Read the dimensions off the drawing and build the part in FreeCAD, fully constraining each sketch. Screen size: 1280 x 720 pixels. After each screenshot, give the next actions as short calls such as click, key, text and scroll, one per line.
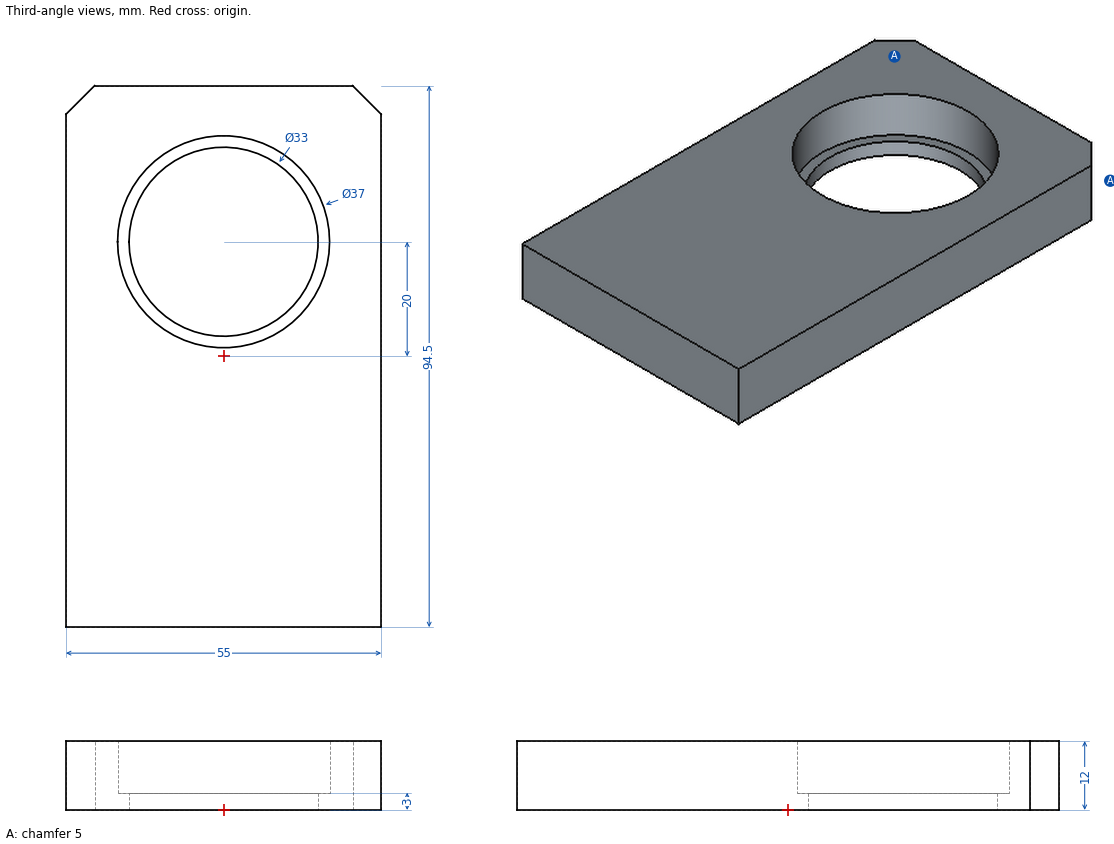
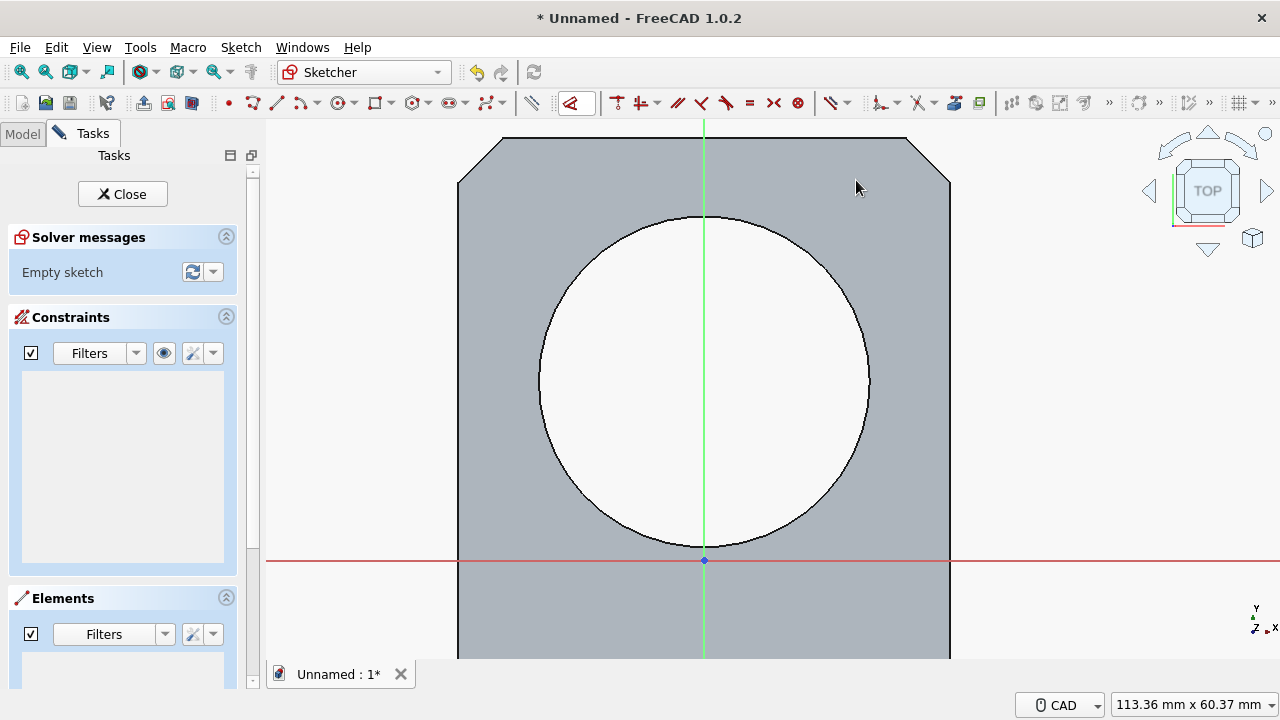
click(338, 104)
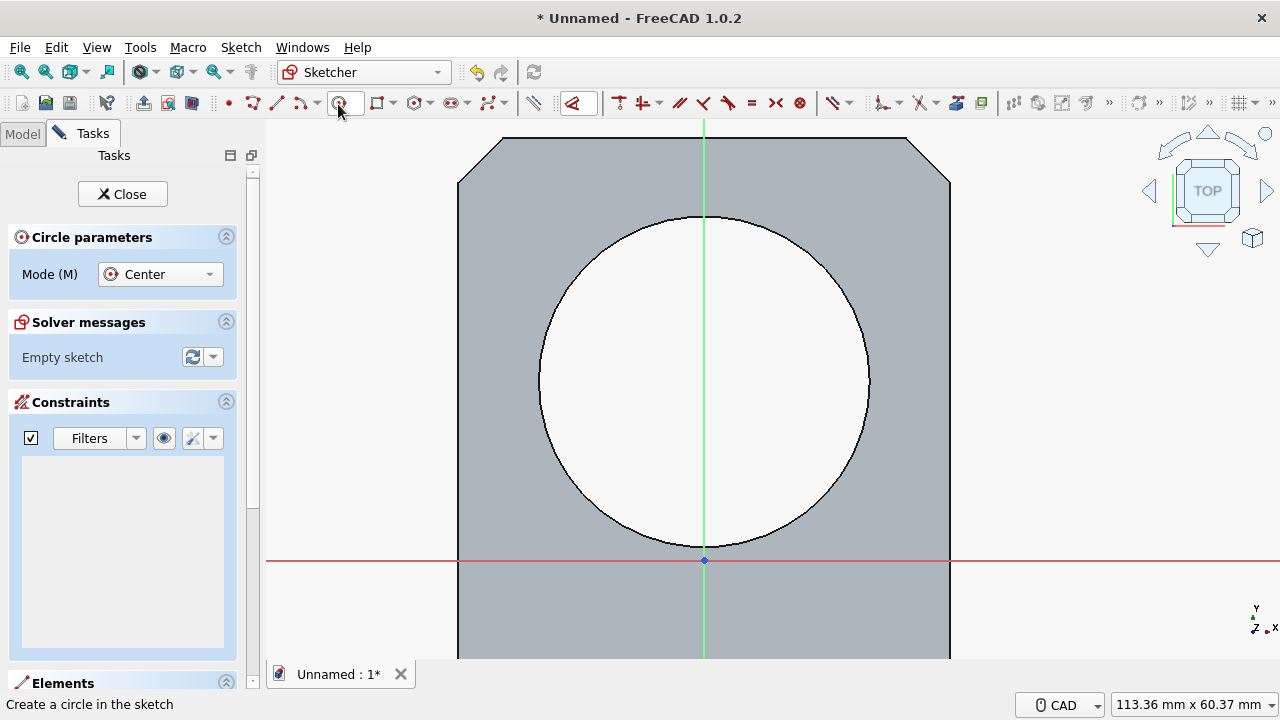
click(704, 382)
click(821, 265)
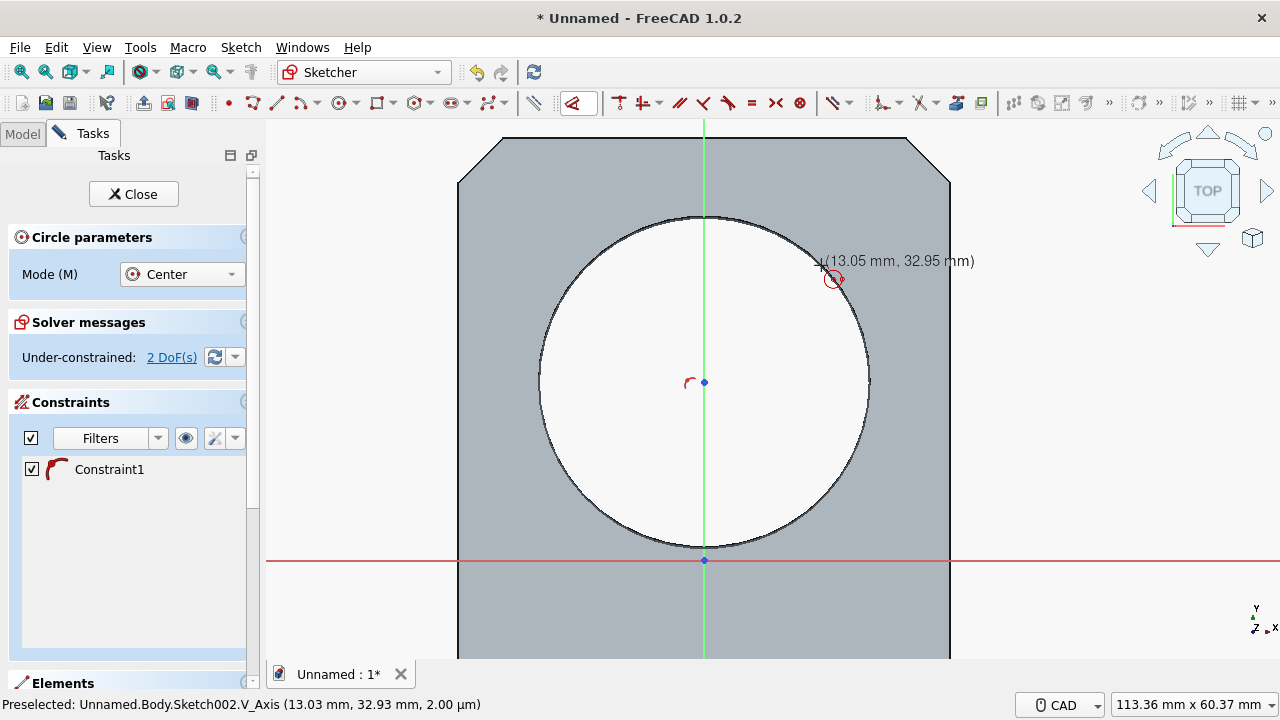
click(704, 383)
click(809, 277)
key(Escape)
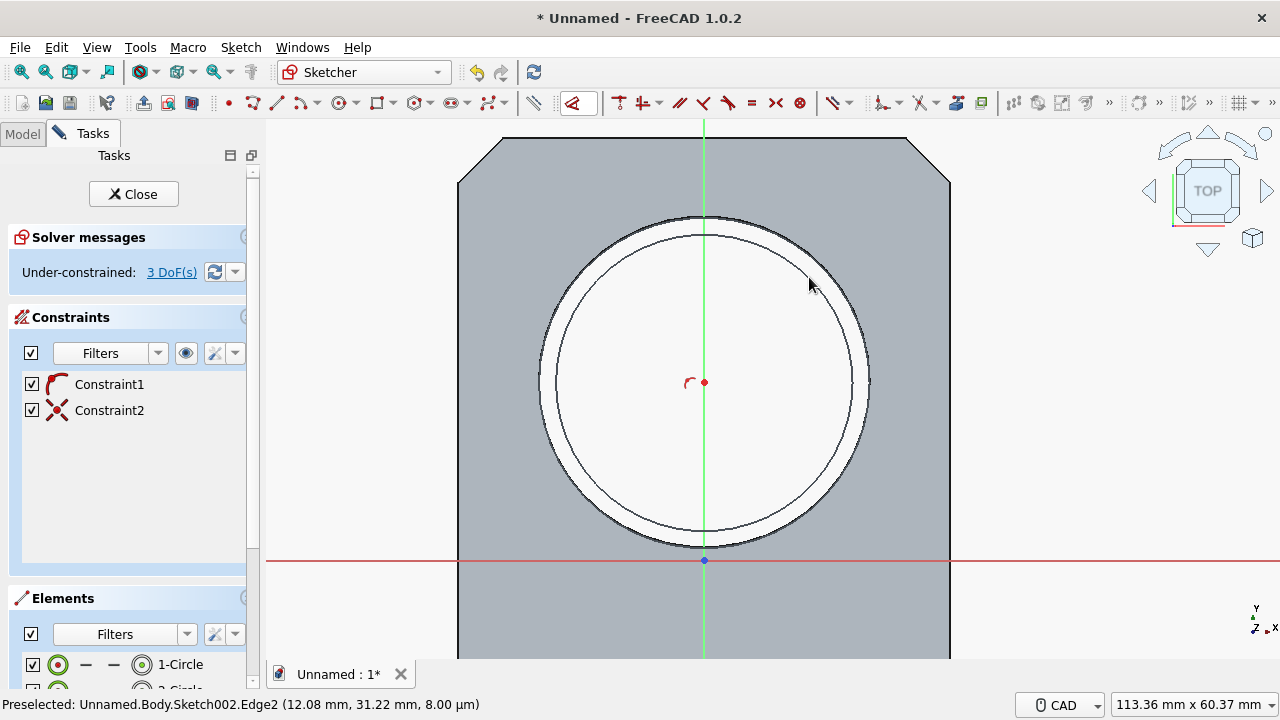
click(821, 266)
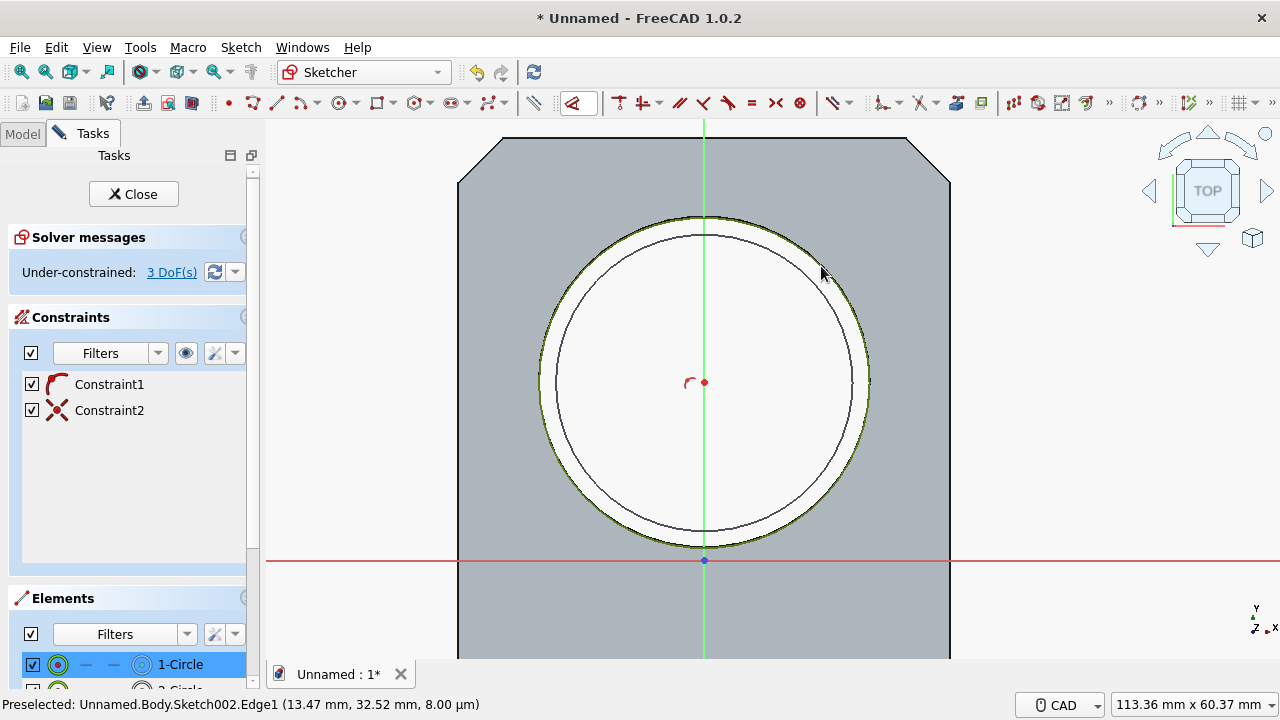
key(k)
key(o)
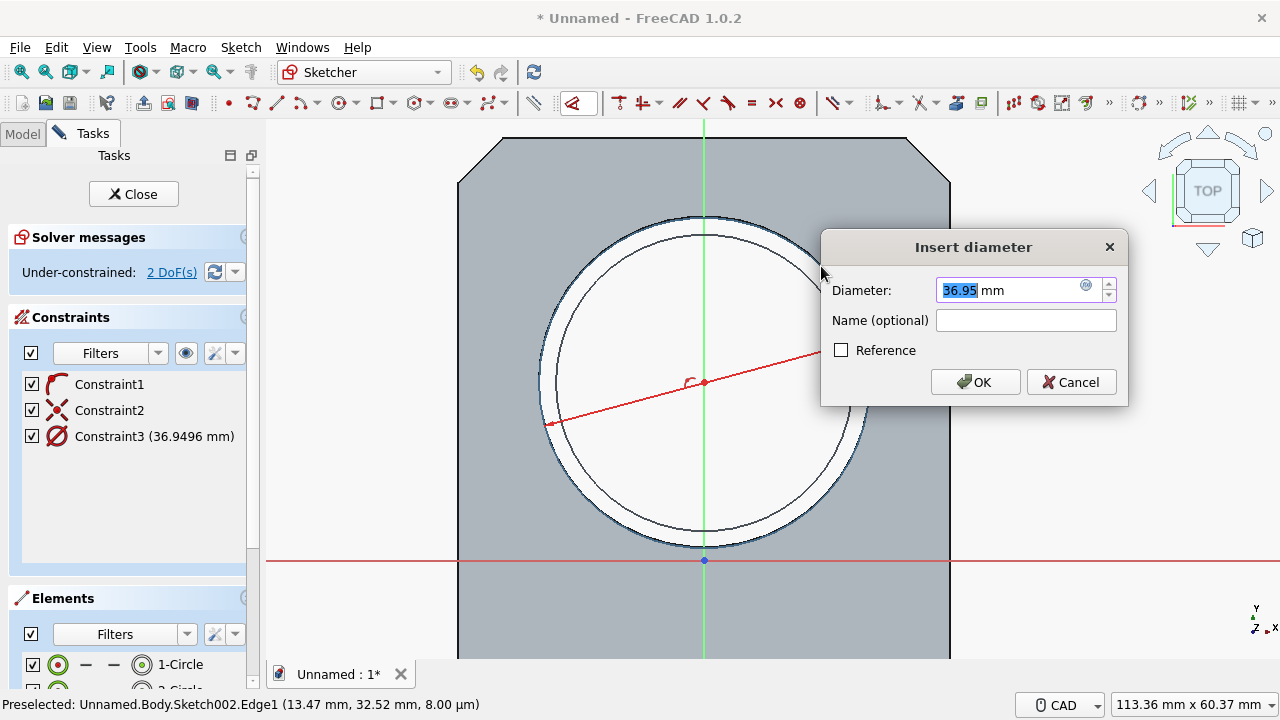
text(37)
key(Return)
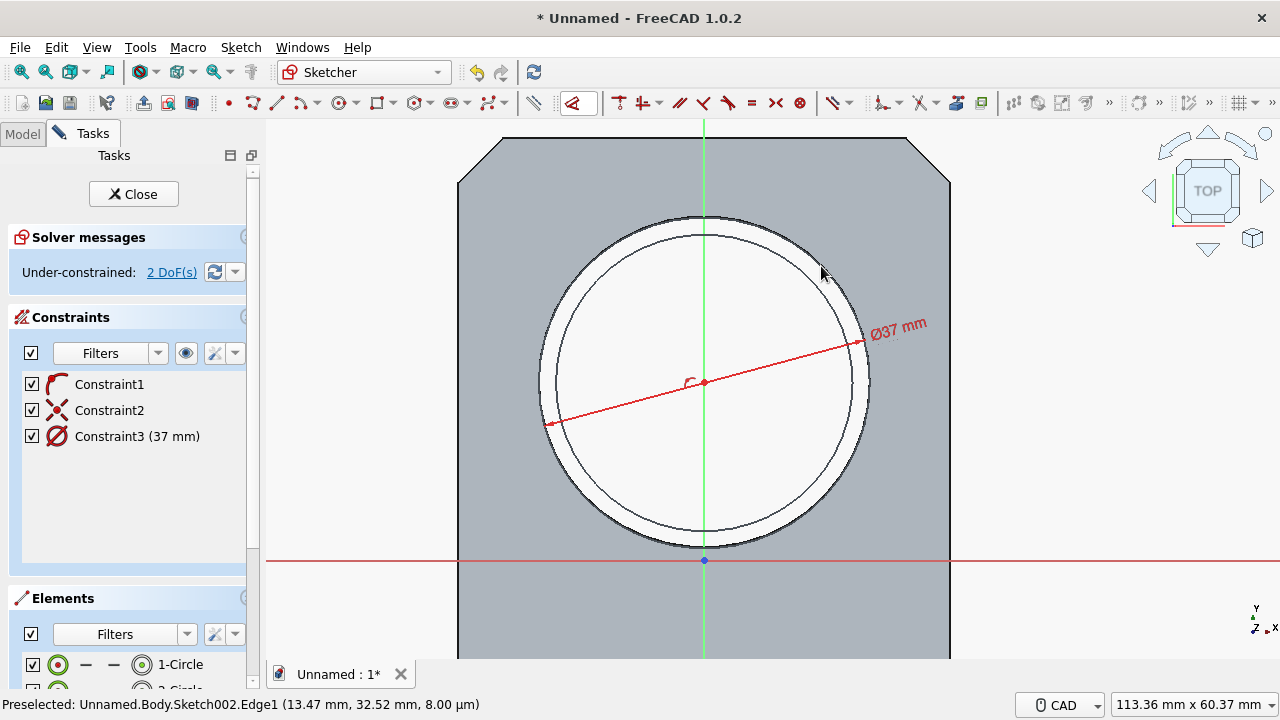
click(809, 278)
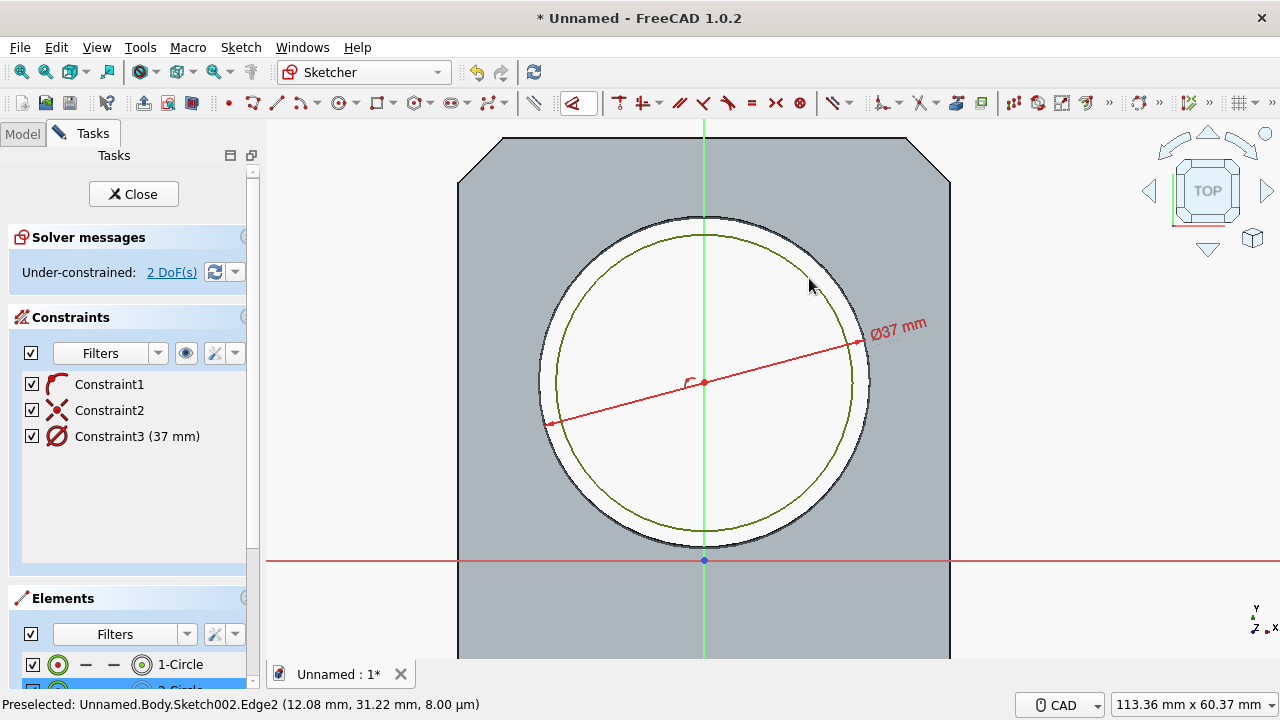
key(k)
key(o)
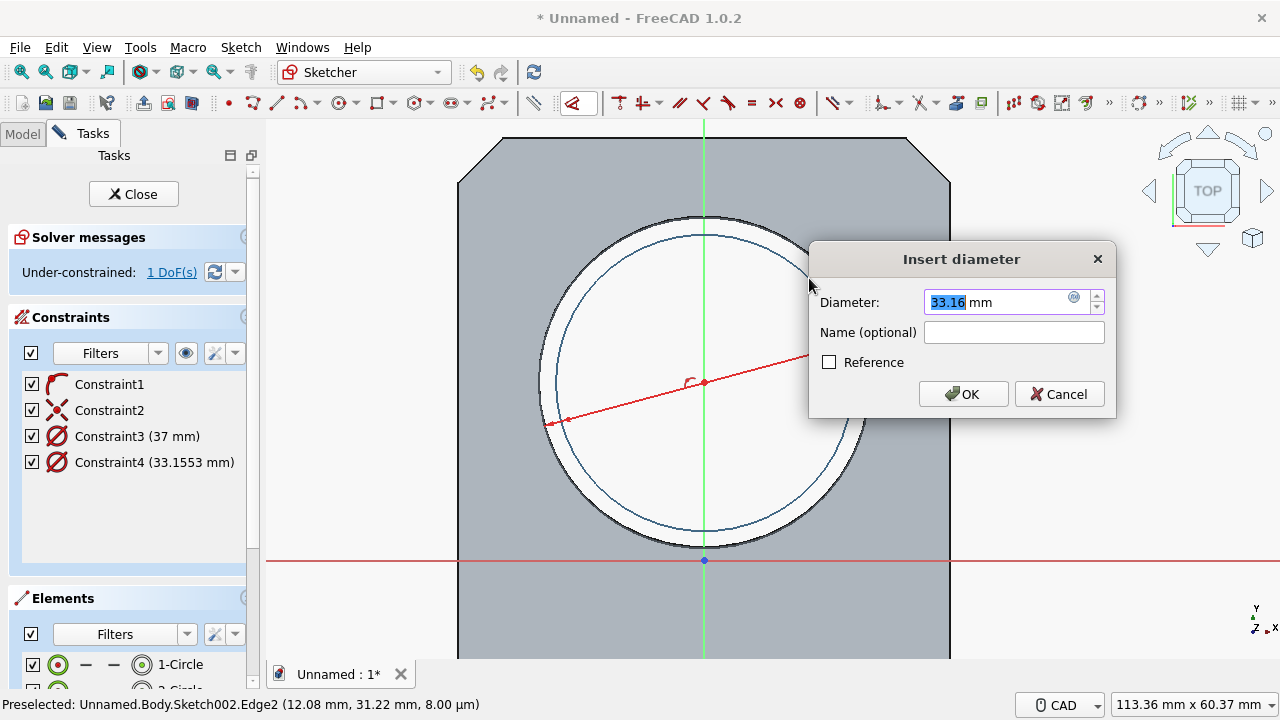
text(33)
key(Return)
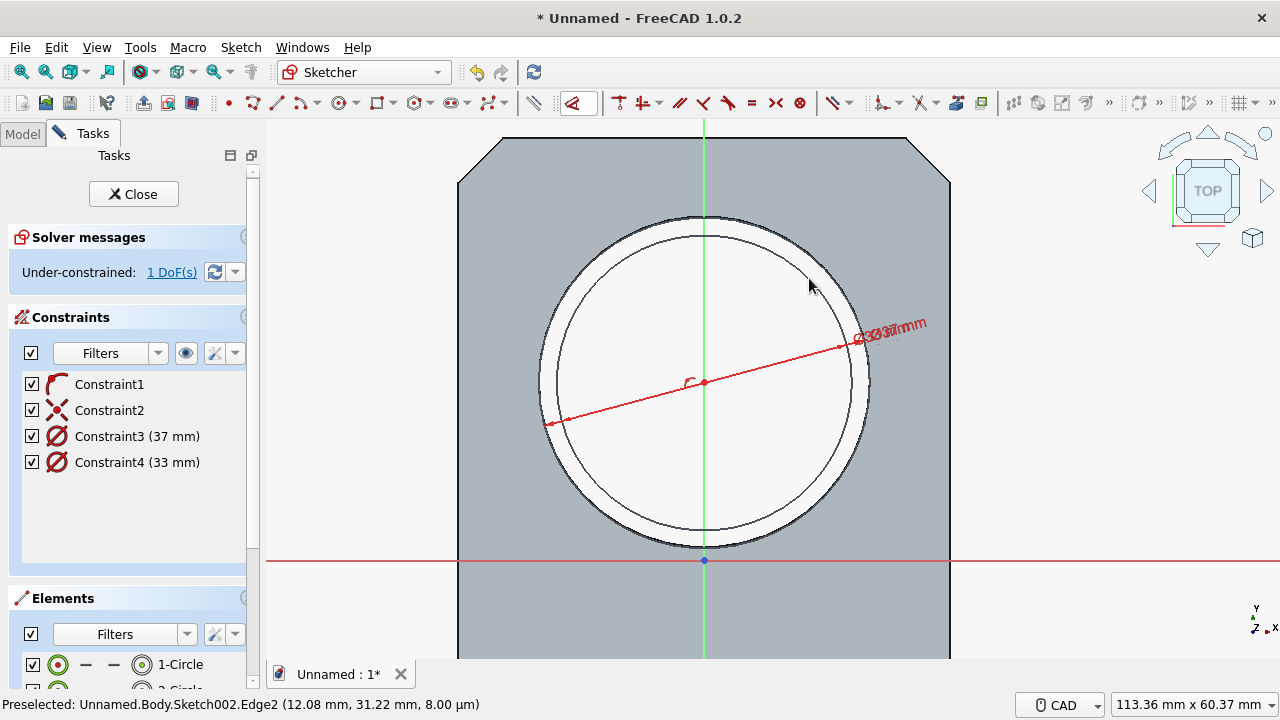
click(704, 383)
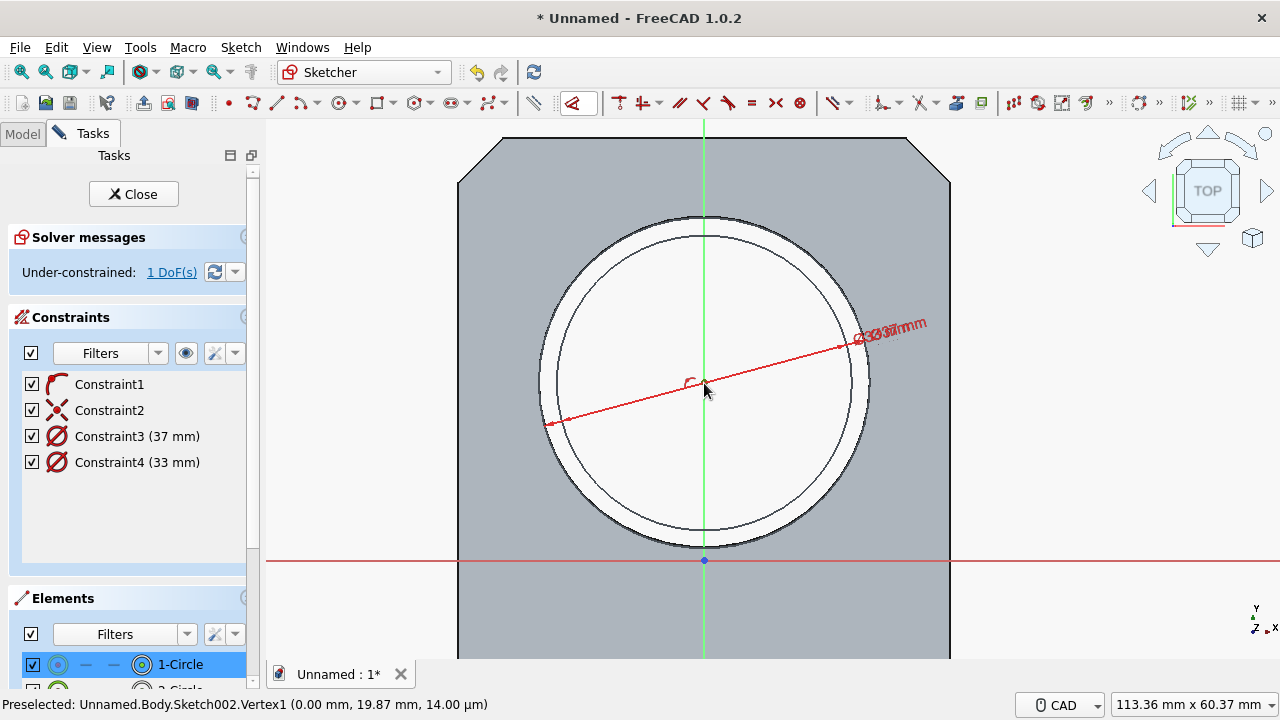
click(592, 104)